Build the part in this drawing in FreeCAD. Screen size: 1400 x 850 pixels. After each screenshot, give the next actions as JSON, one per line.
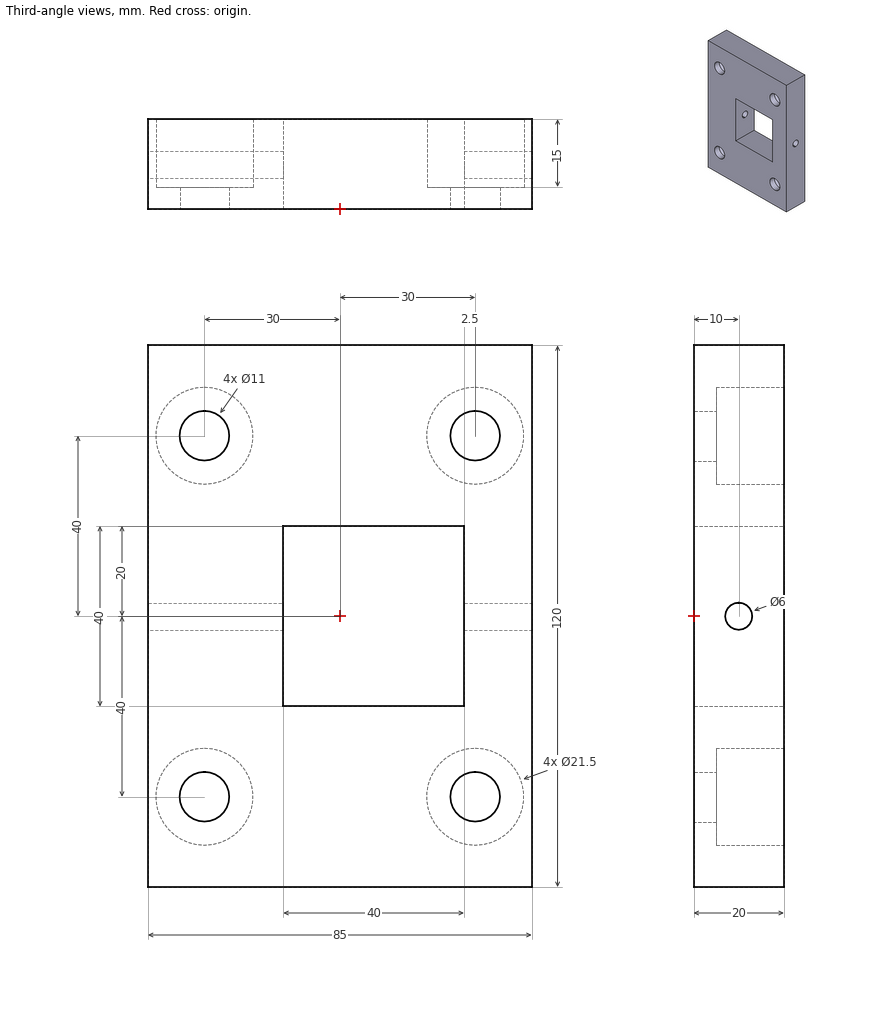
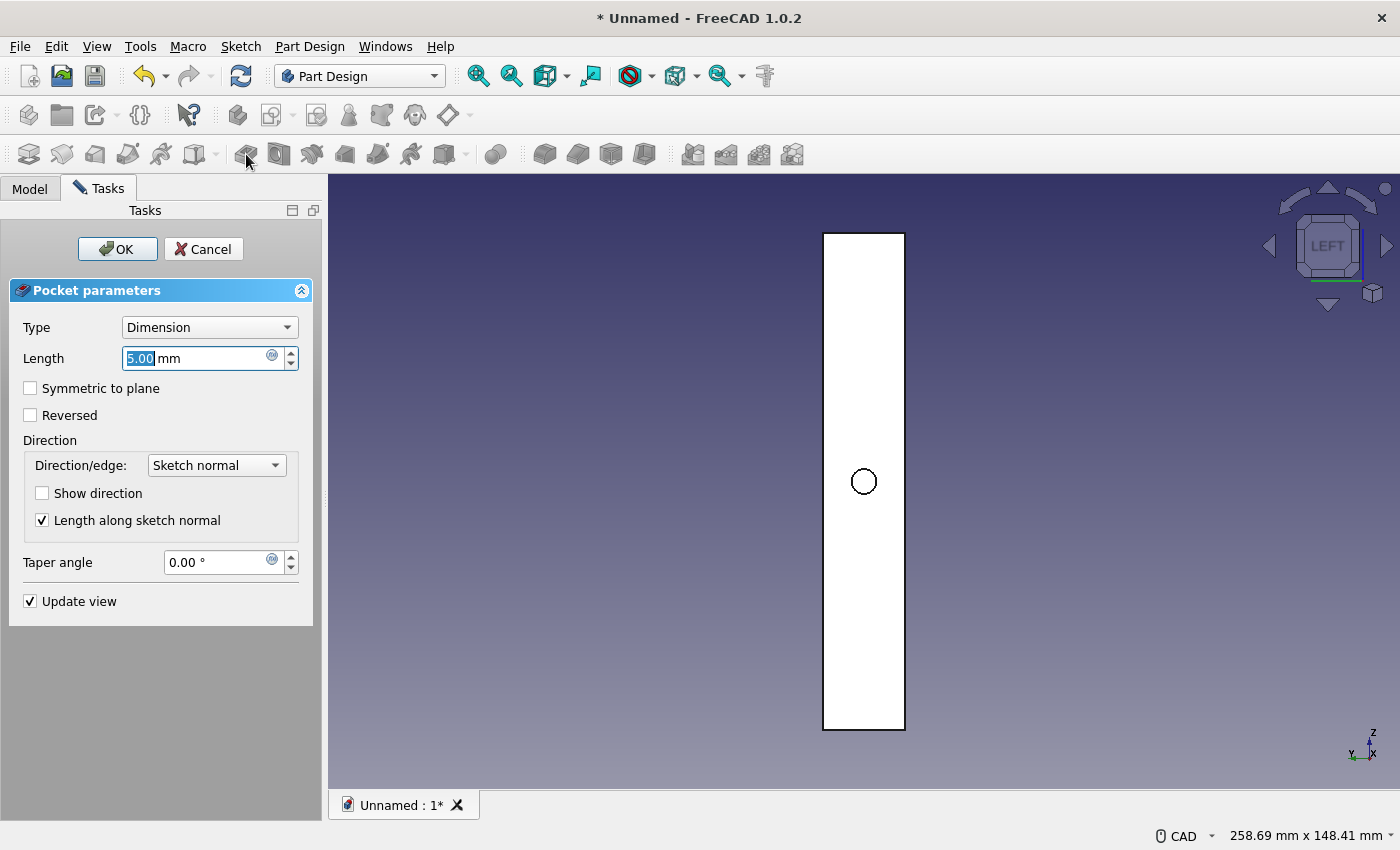
{"action": "left_click", "coordinate": [210, 328]}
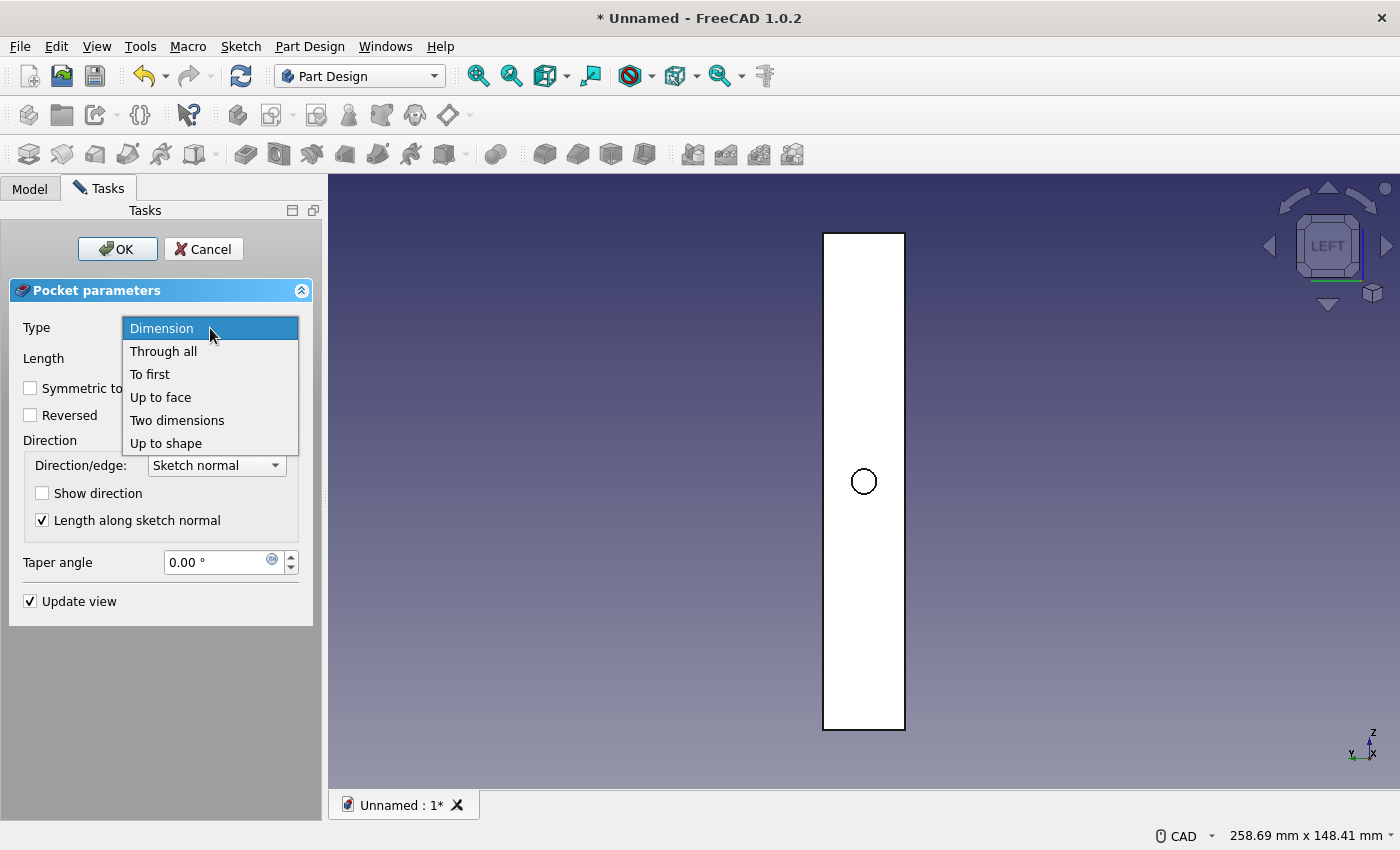
{"action": "left_click", "coordinate": [208, 352]}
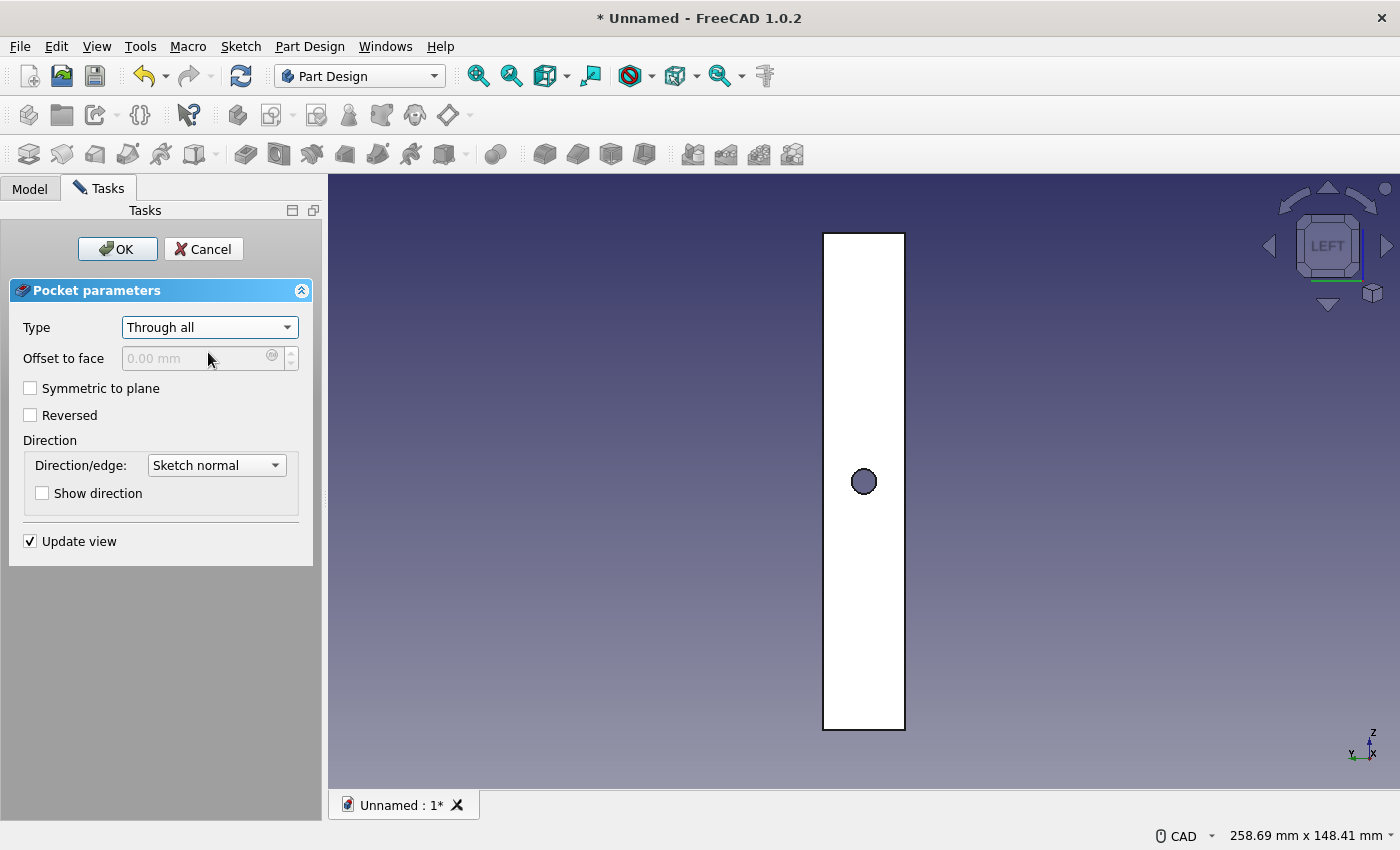
{"action": "left_click", "coordinate": [118, 249]}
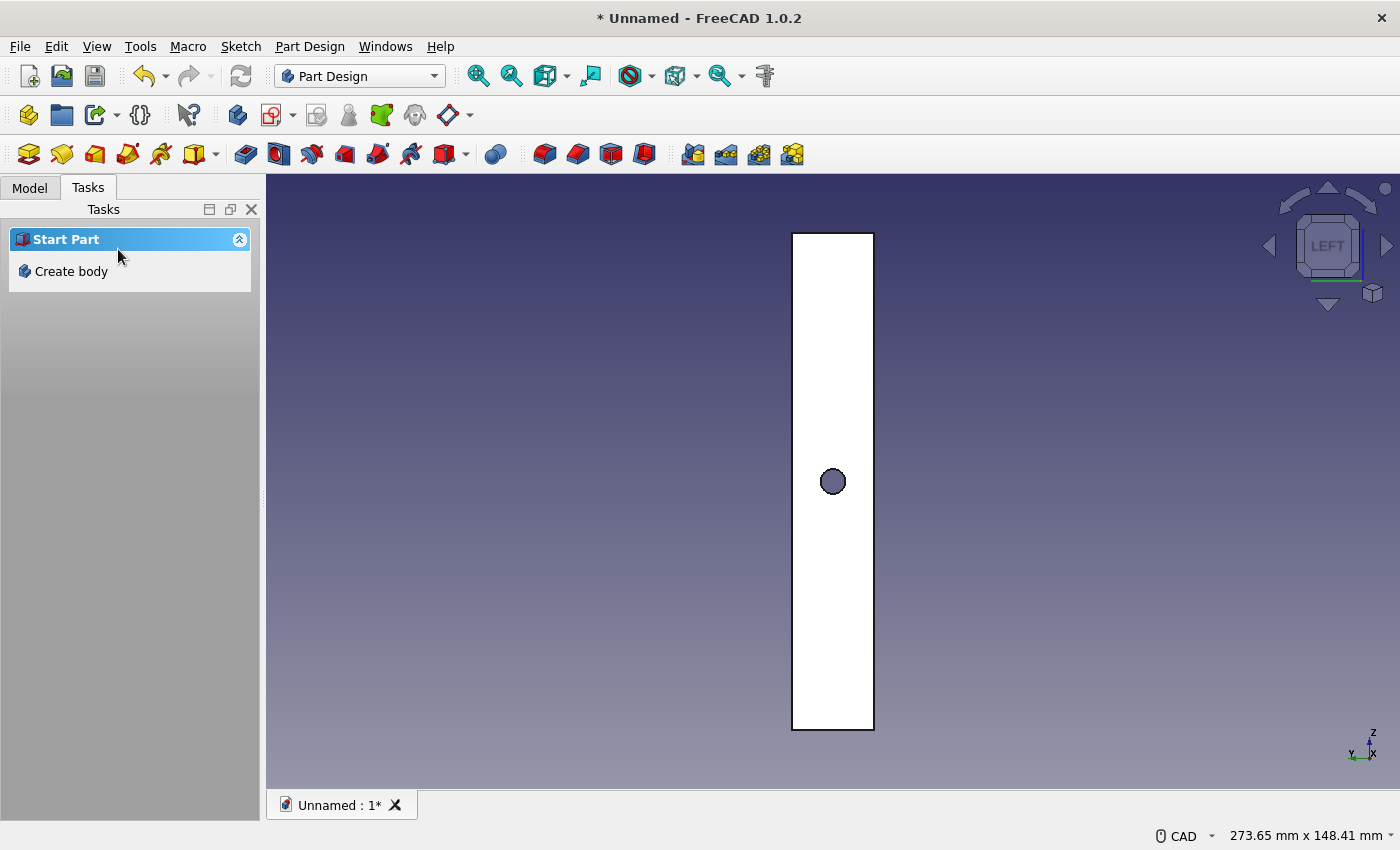
{"action": "key", "text": "0"}